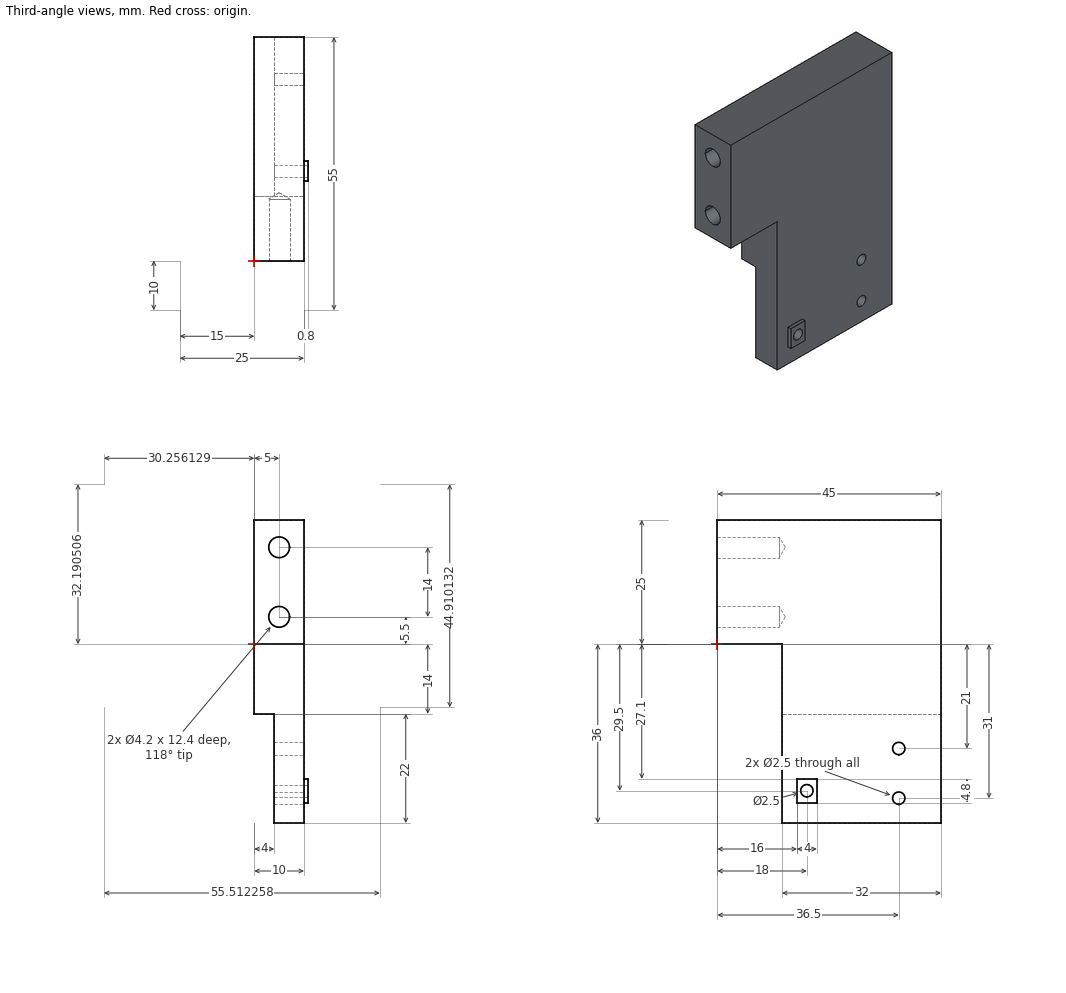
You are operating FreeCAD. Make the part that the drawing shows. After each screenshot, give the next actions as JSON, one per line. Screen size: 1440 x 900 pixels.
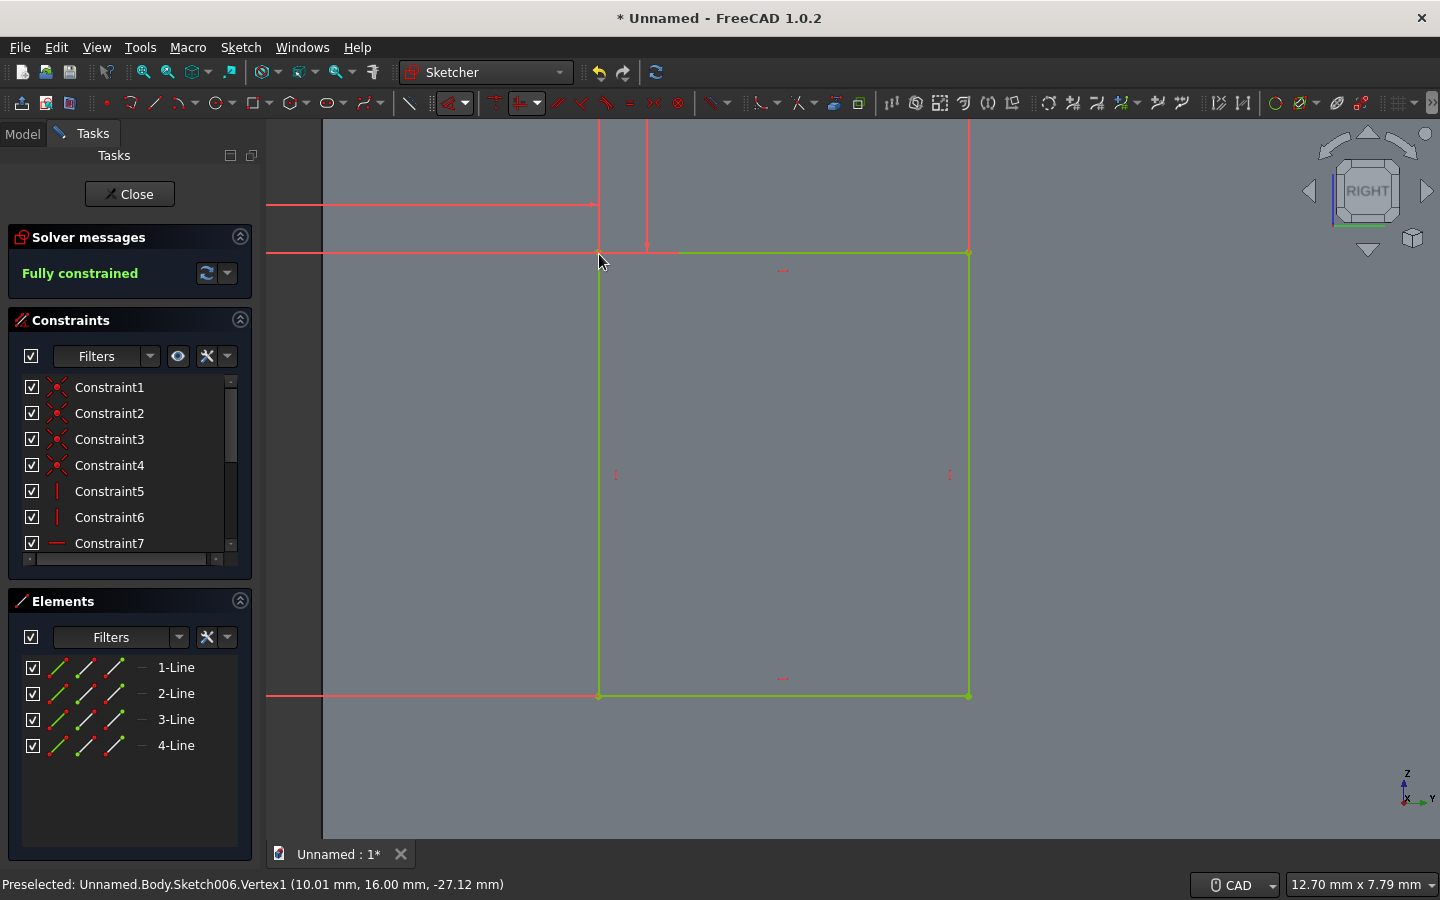
{"action": "left_click", "coordinate": [130, 194]}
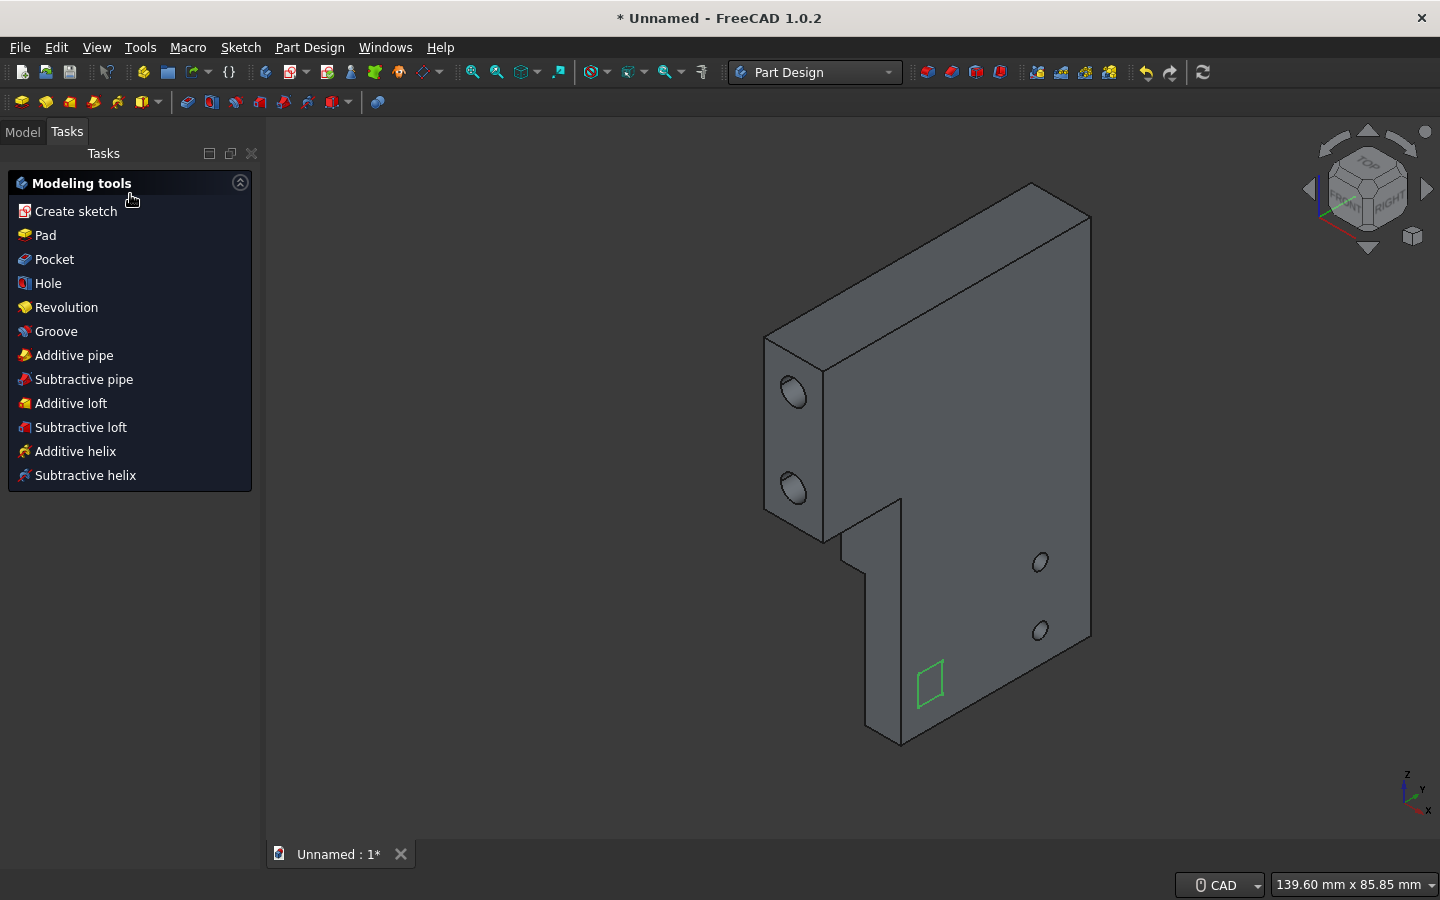
{"action": "left_click", "coordinate": [22, 102]}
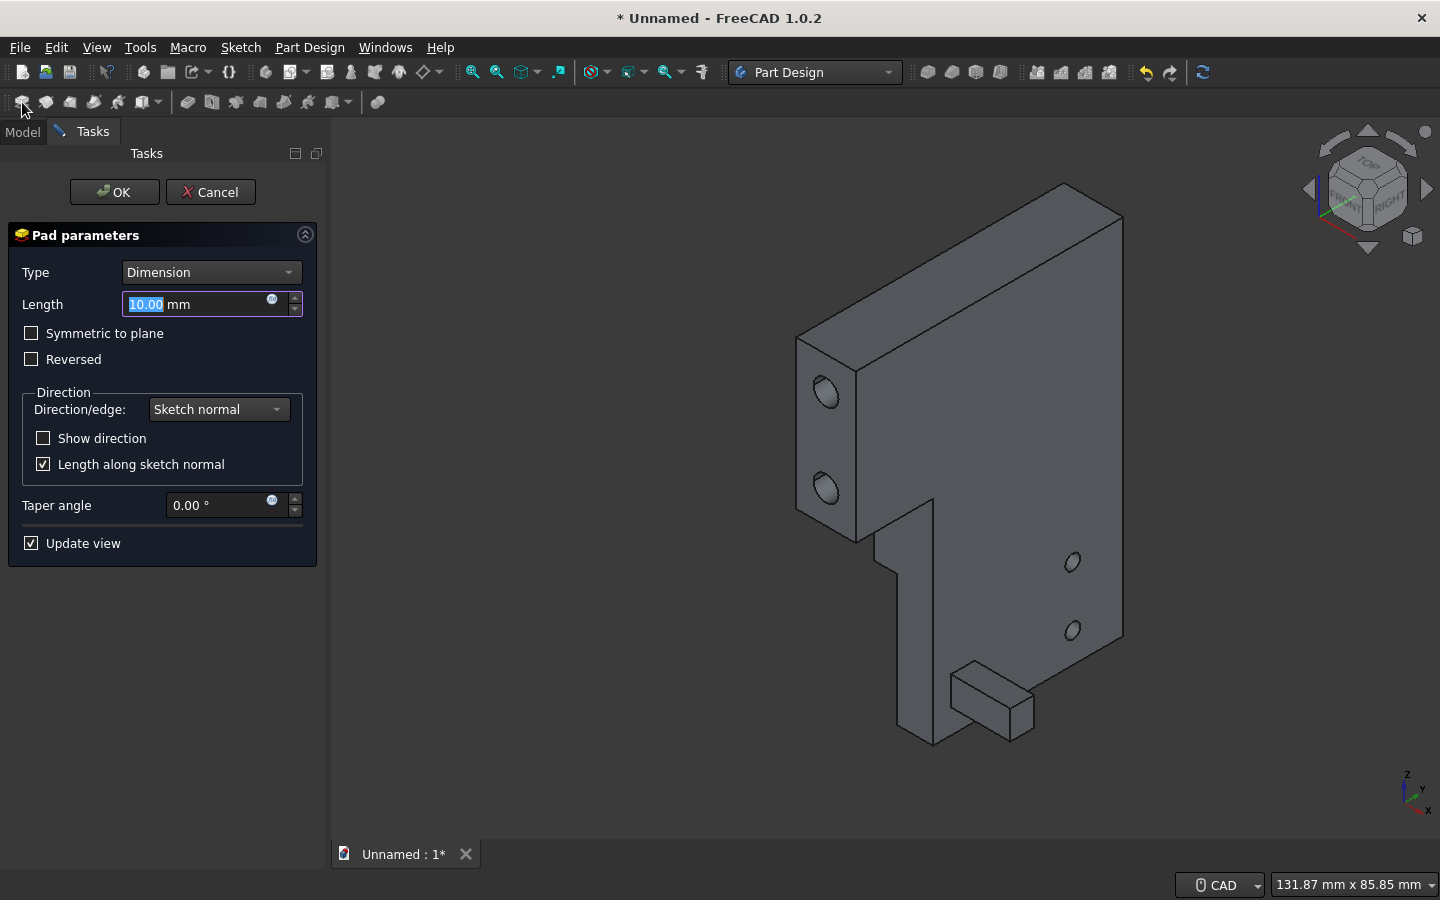
{"action": "type", "text": "0.8"}
{"action": "key", "text": "Tab"}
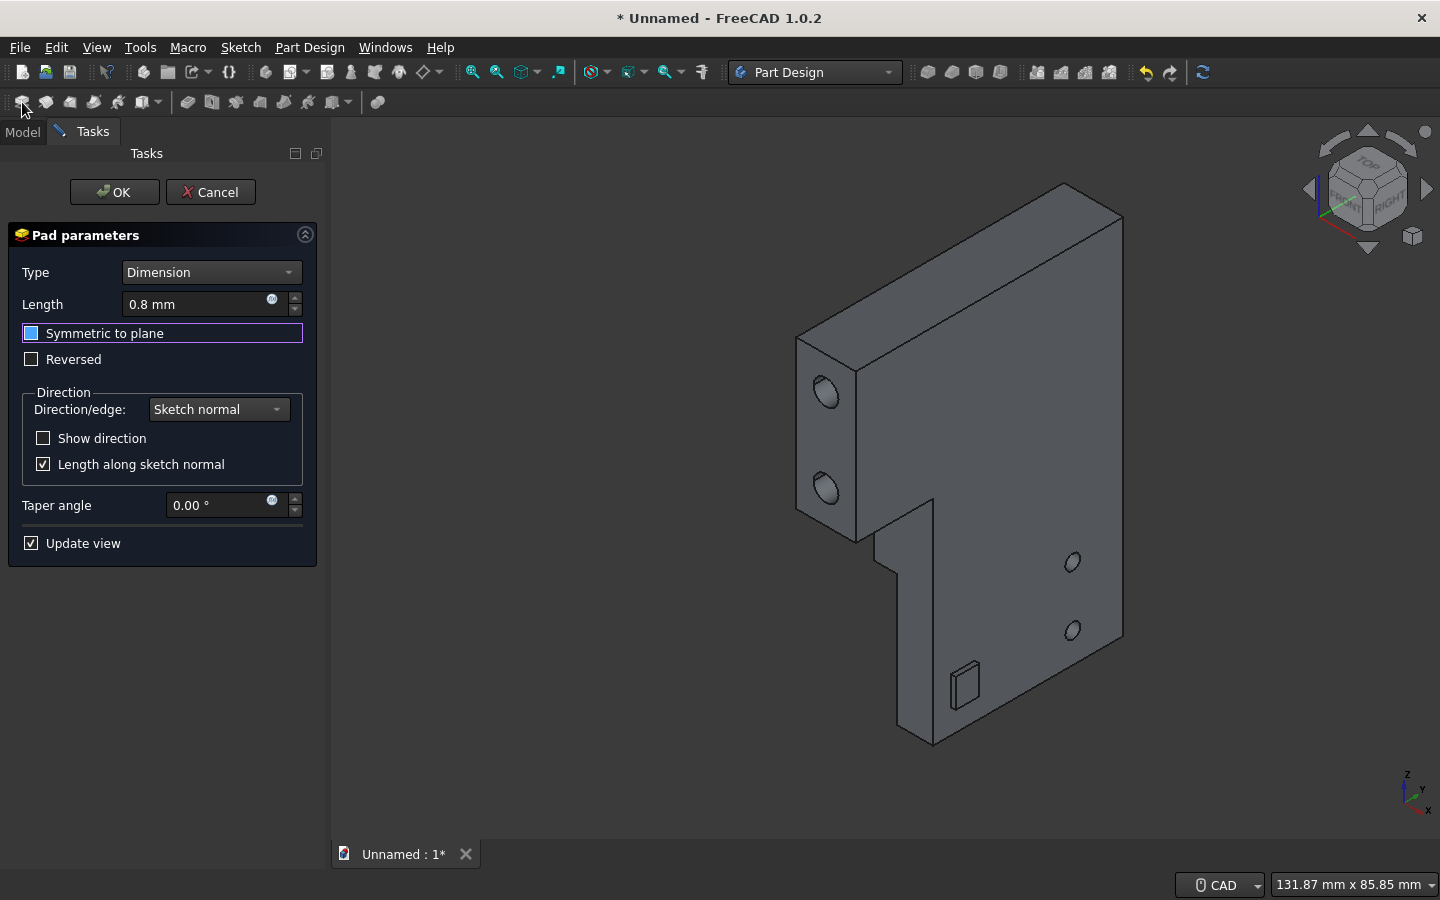
{"action": "left_click", "coordinate": [115, 192]}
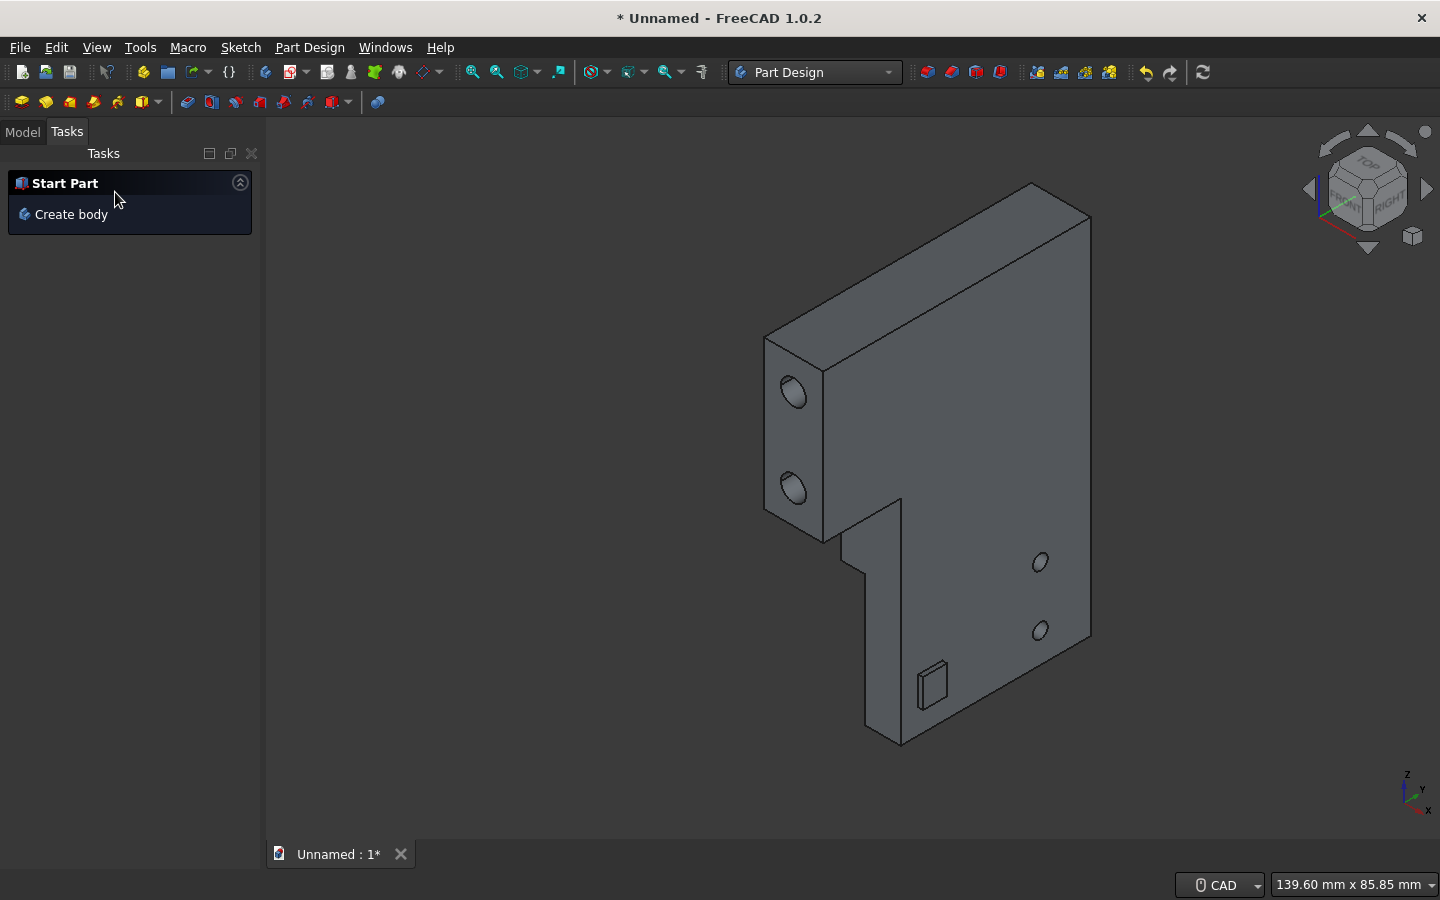
{"action": "key", "text": "6"}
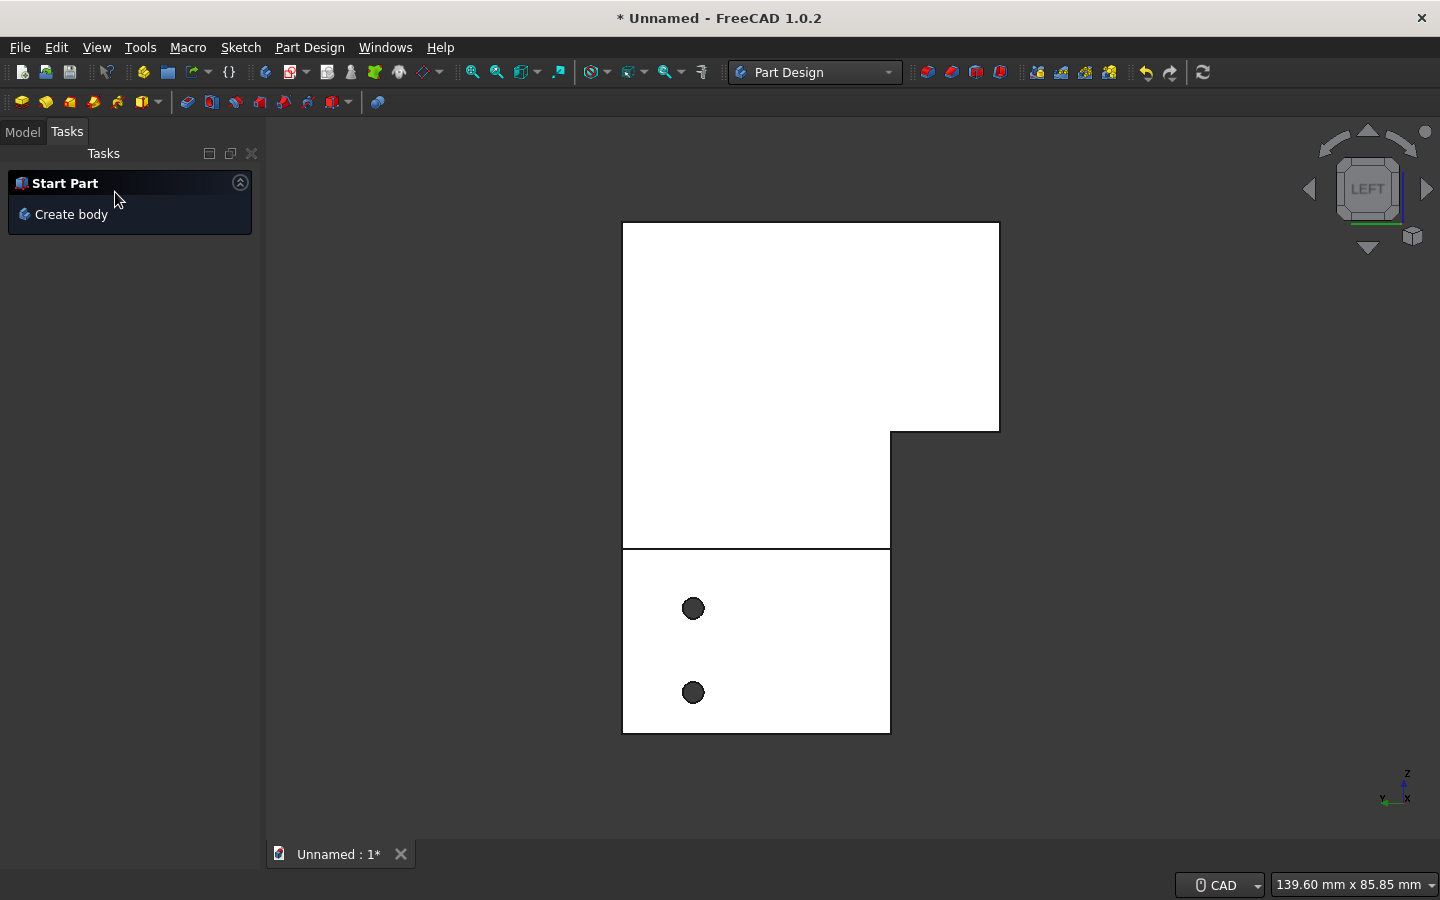
{"action": "left_click", "coordinate": [757, 384]}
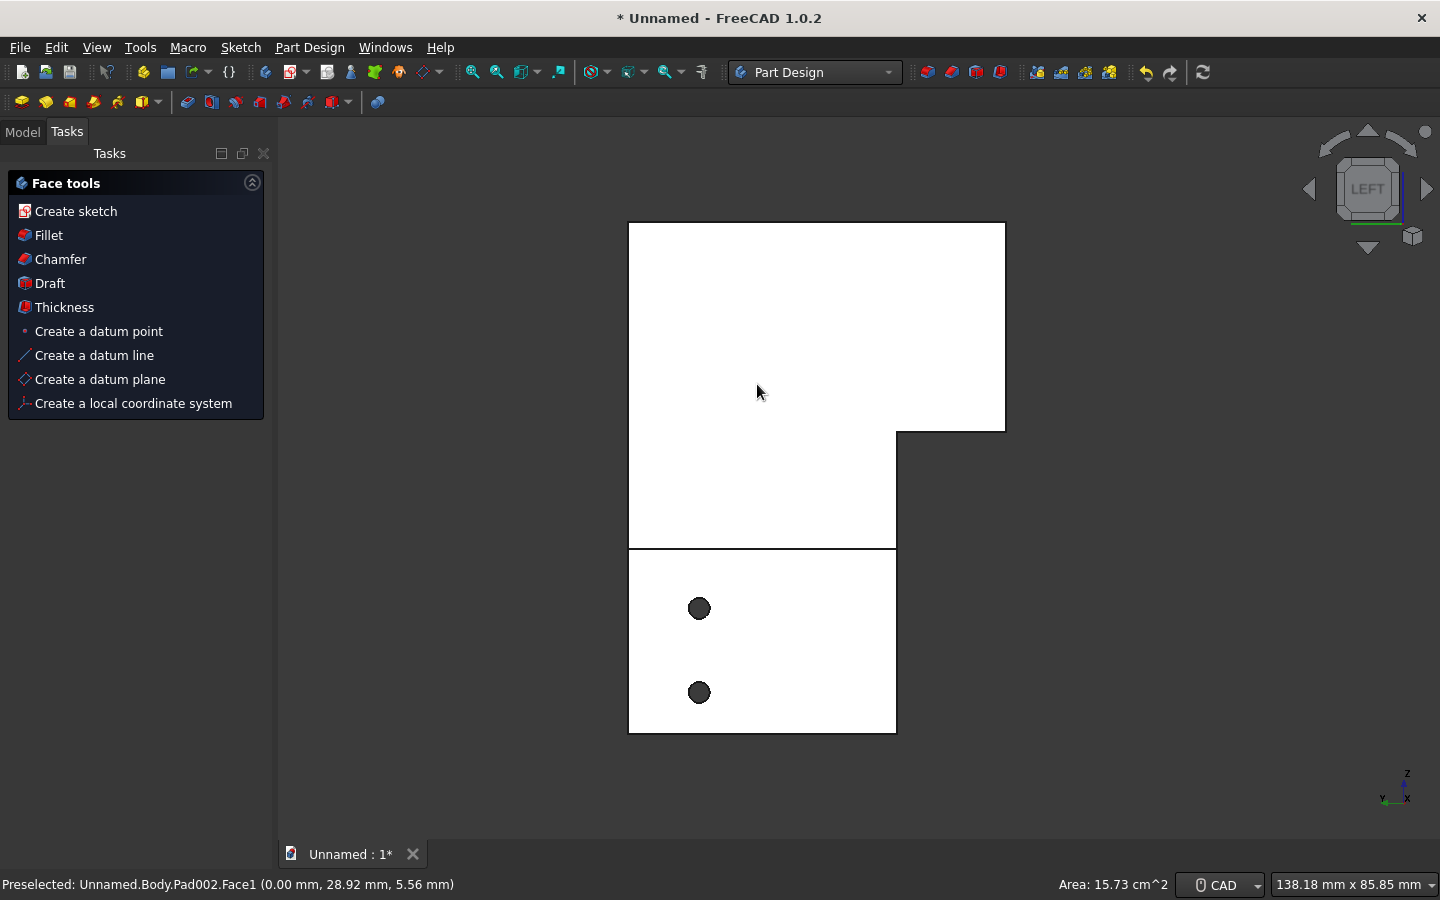
{"action": "left_click", "coordinate": [290, 72]}